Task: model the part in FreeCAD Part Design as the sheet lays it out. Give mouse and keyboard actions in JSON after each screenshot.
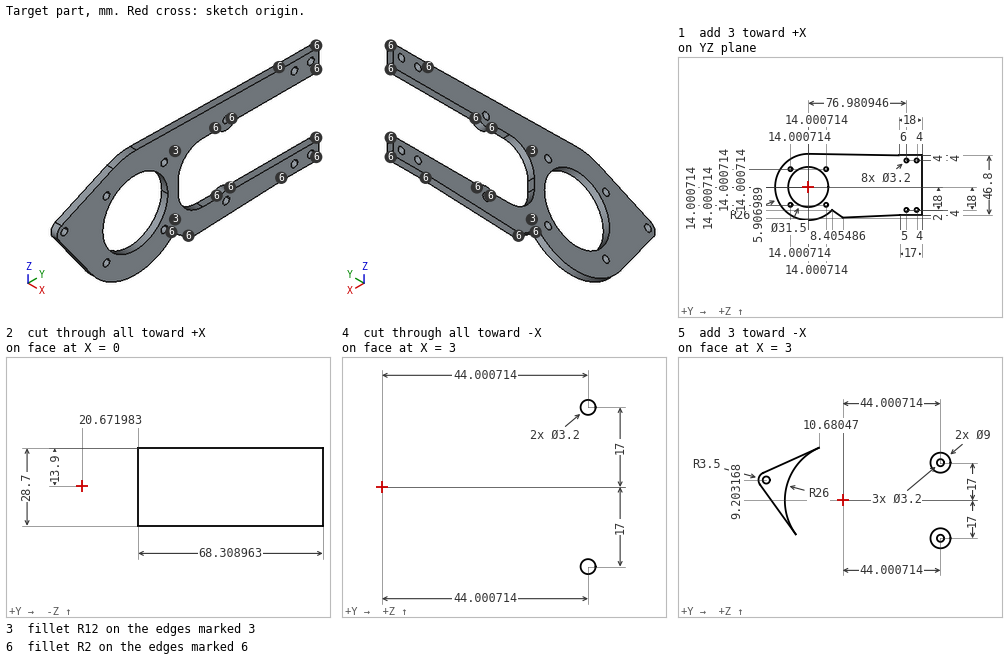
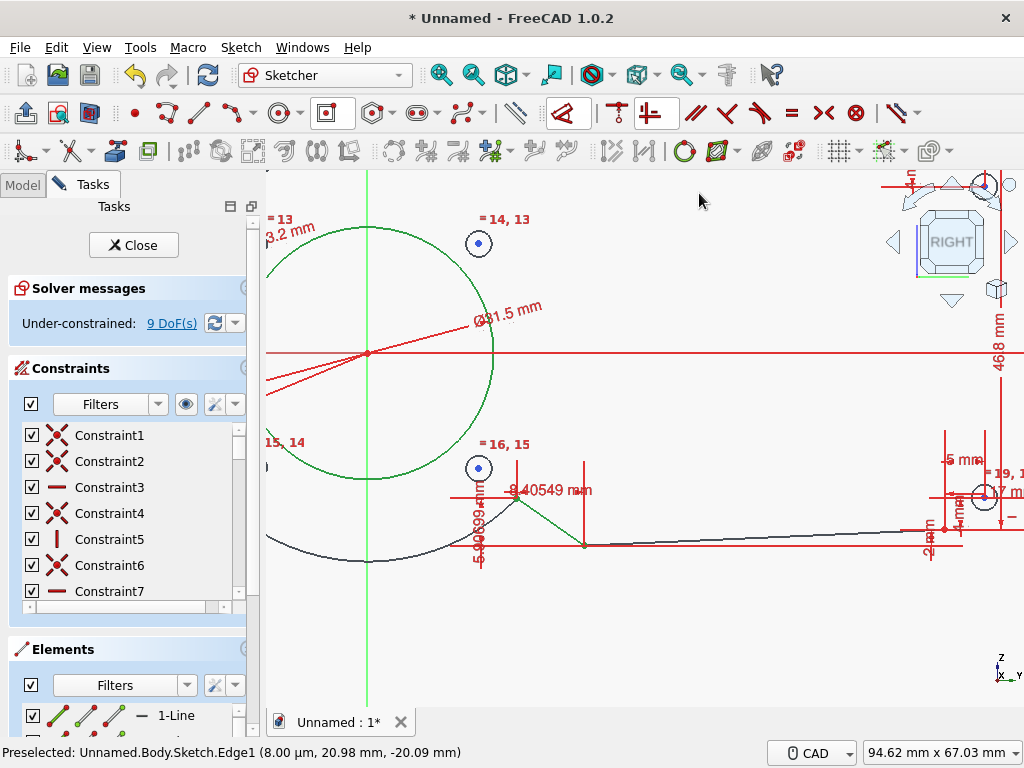
{"action": "scroll", "coordinate": [535, 514], "scroll_direction": "down", "scroll_amount": 4}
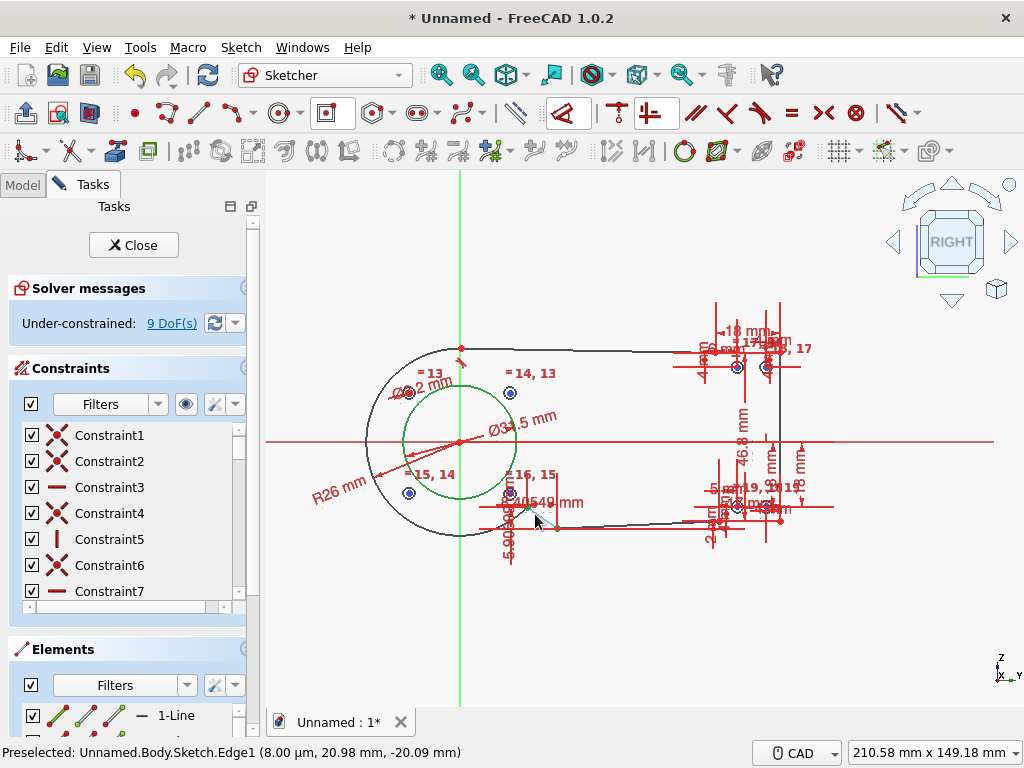
{"action": "left_click", "coordinate": [409, 393]}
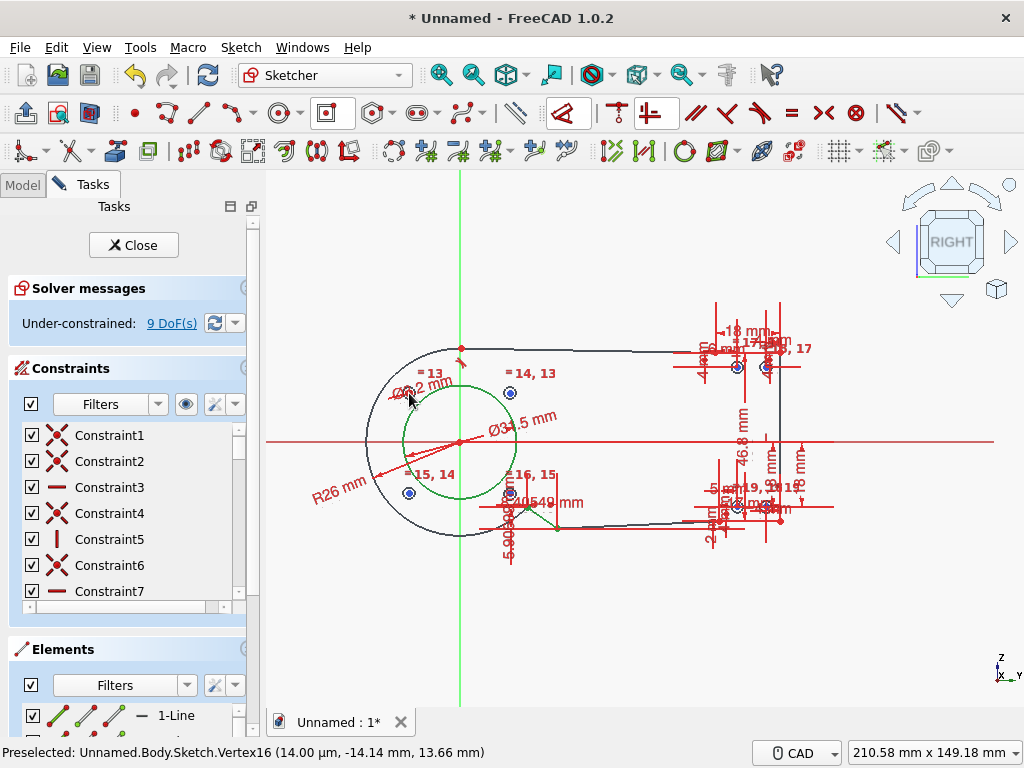
{"action": "left_click", "coordinate": [586, 114]}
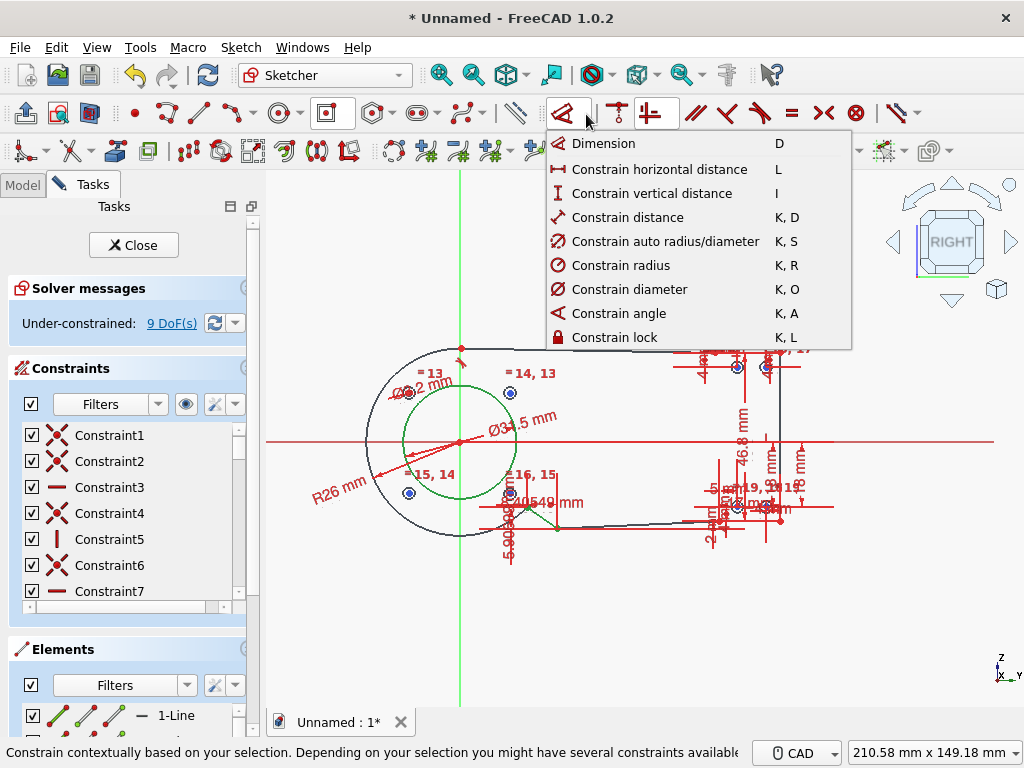
{"action": "left_click", "coordinate": [699, 169]}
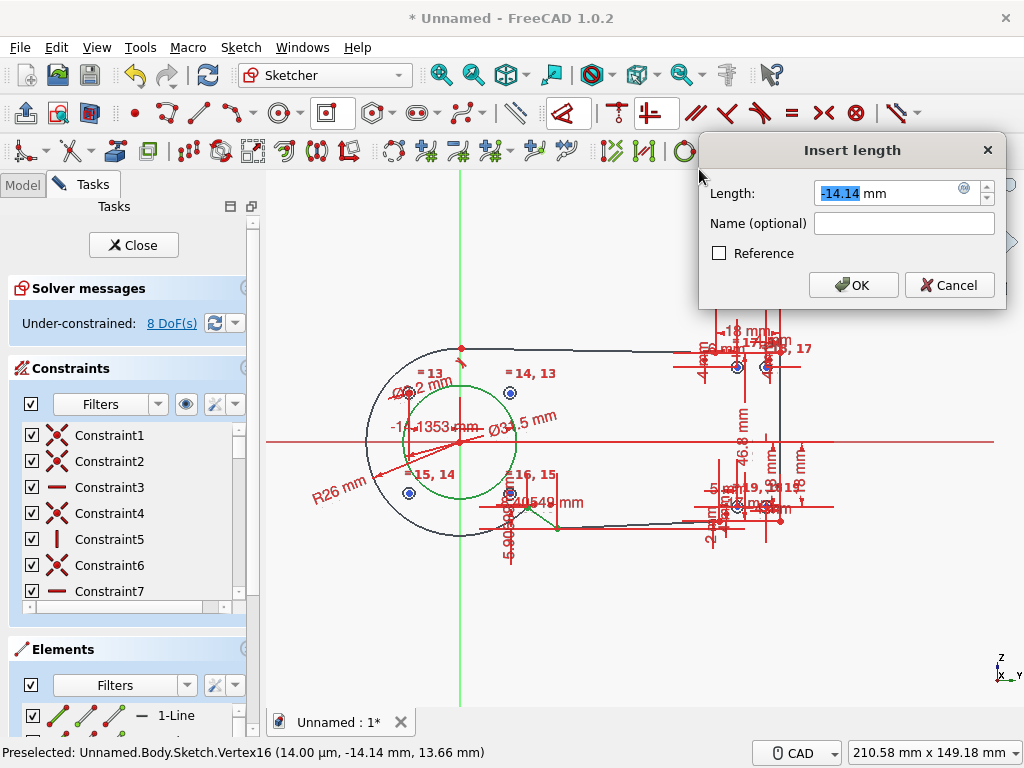
{"action": "type", "text": "-14.000714"}
{"action": "key", "text": "Return"}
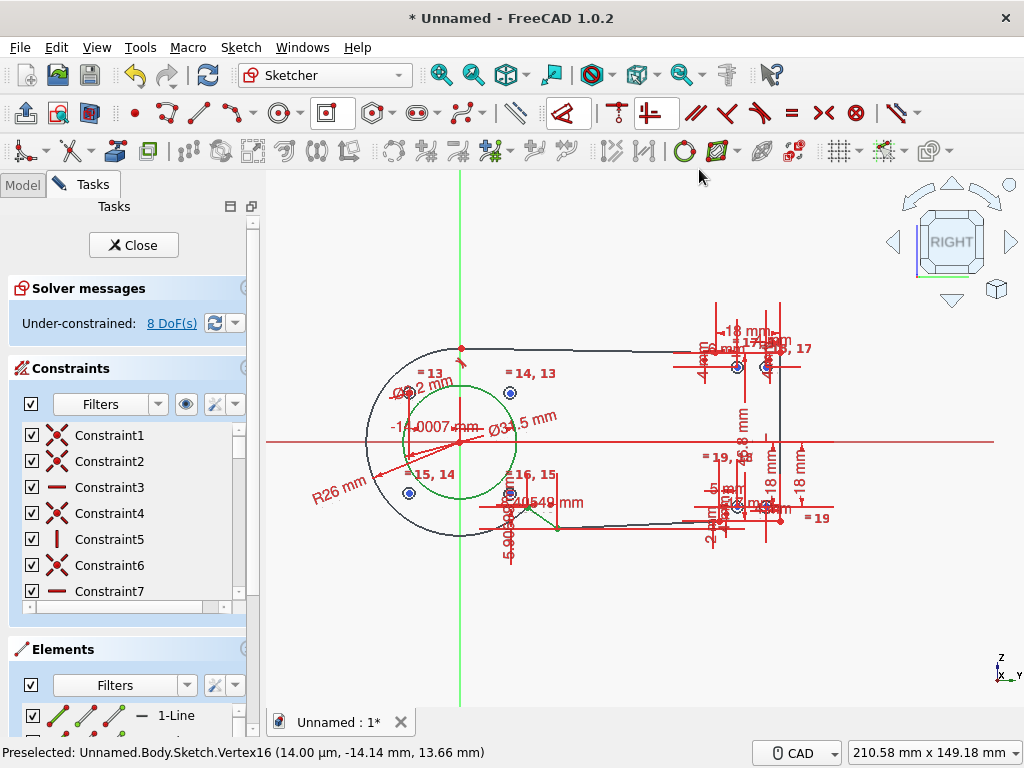
{"action": "left_click", "coordinate": [409, 393]}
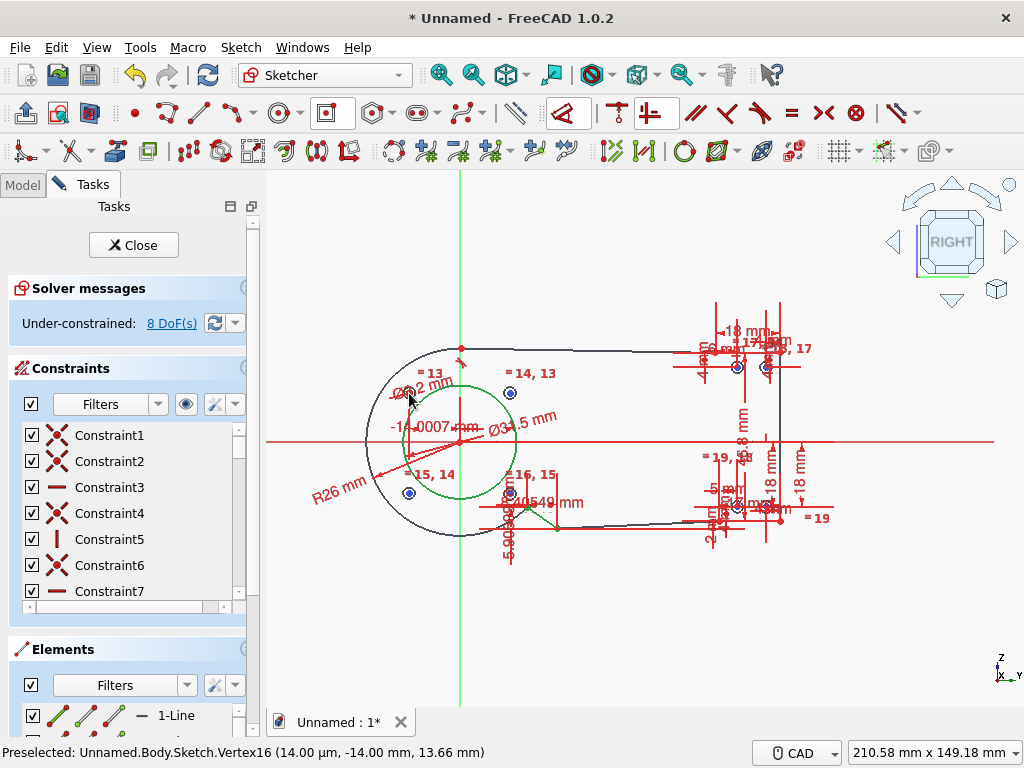
{"action": "key", "text": "i"}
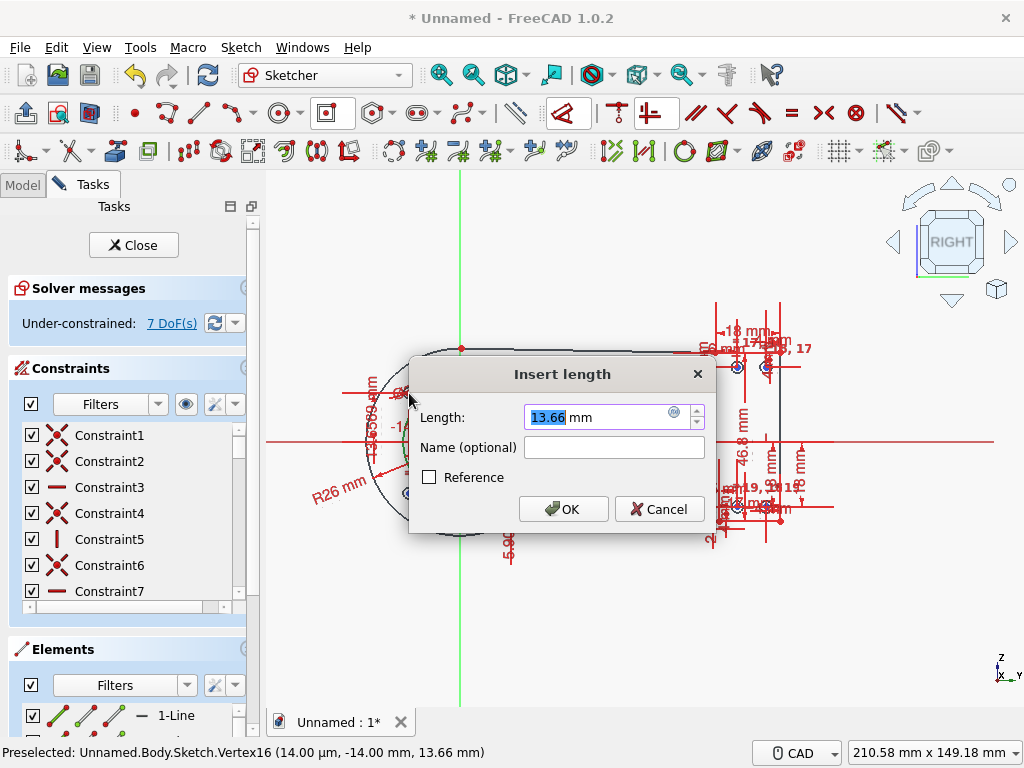
{"action": "type", "text": "14.000714"}
{"action": "key", "text": "Return"}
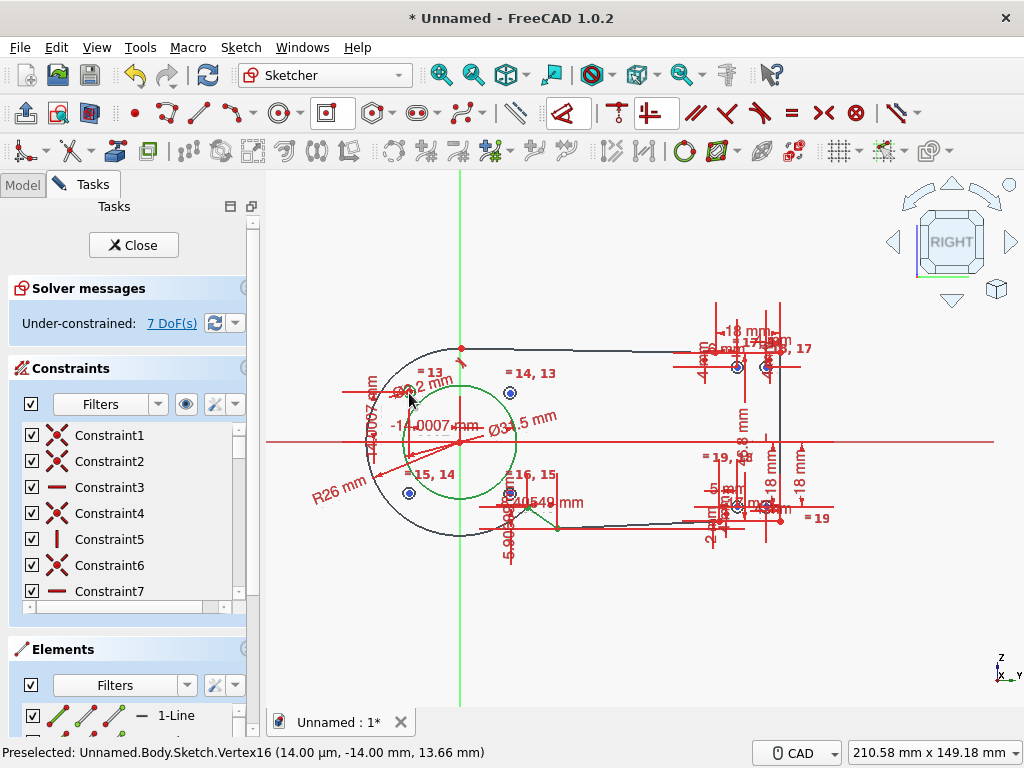
{"action": "left_click", "coordinate": [510, 393]}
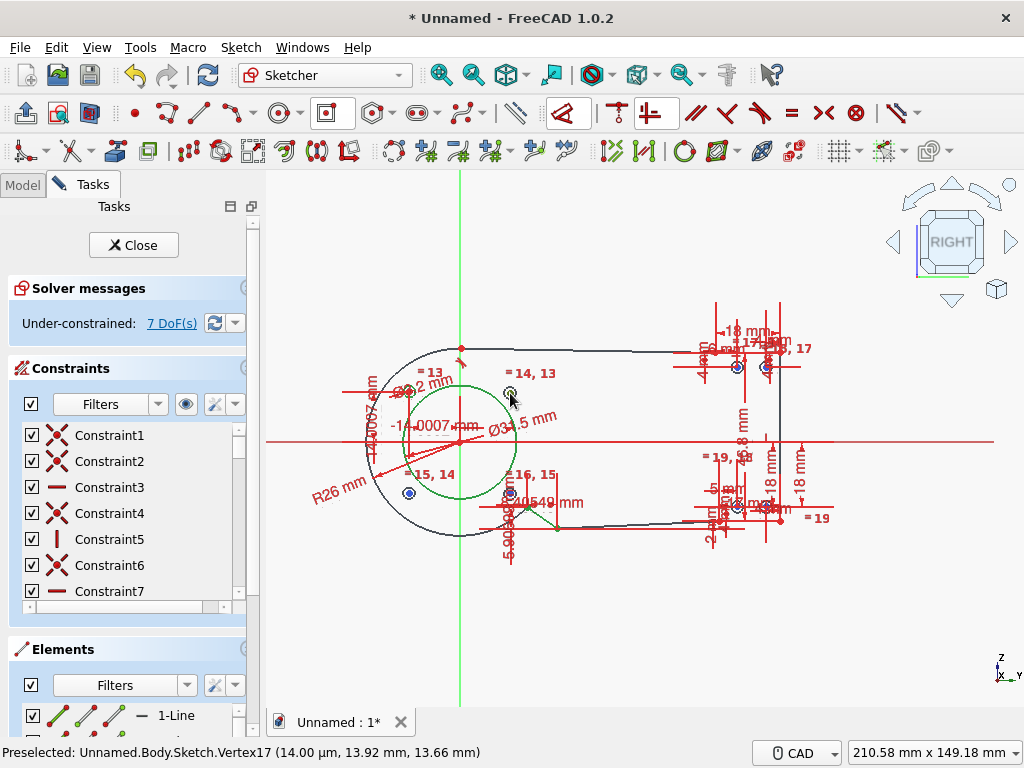
{"action": "left_click", "coordinate": [586, 114]}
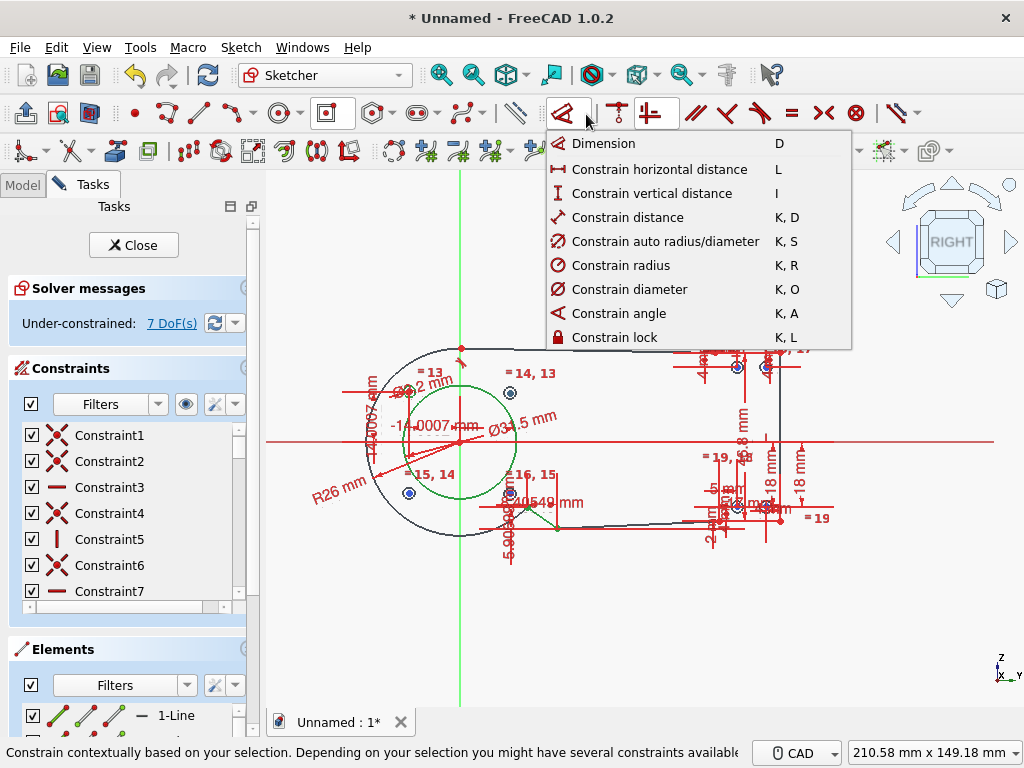
{"action": "left_click", "coordinate": [699, 169]}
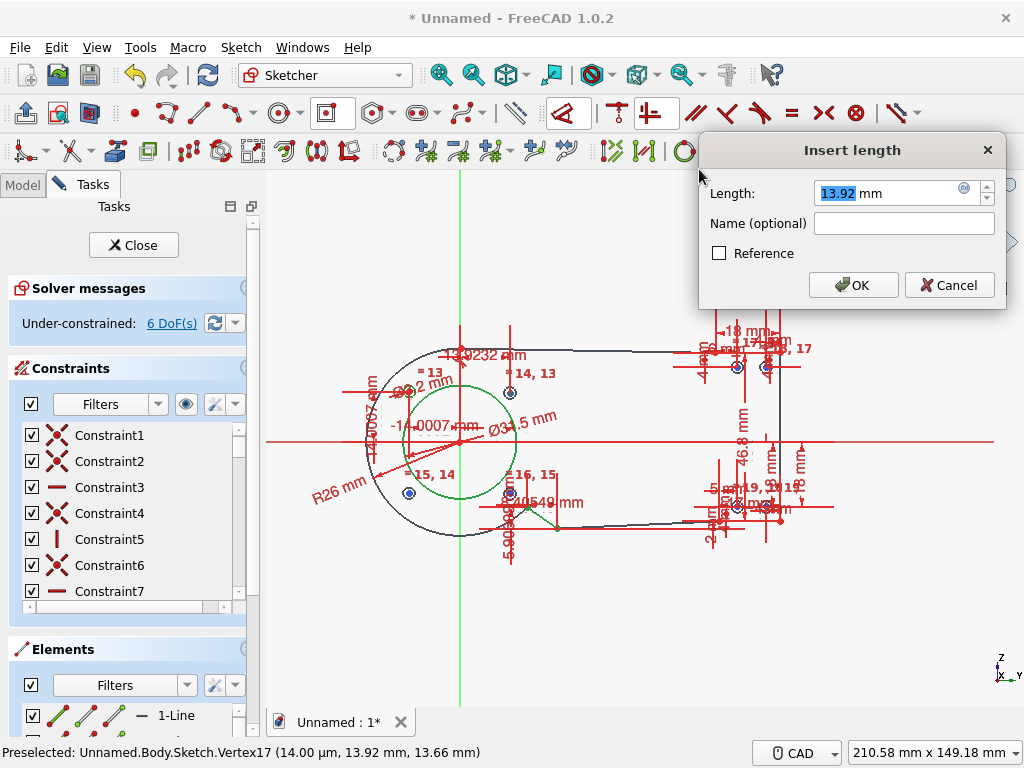
{"action": "type", "text": "14.000714"}
{"action": "key", "text": "Return"}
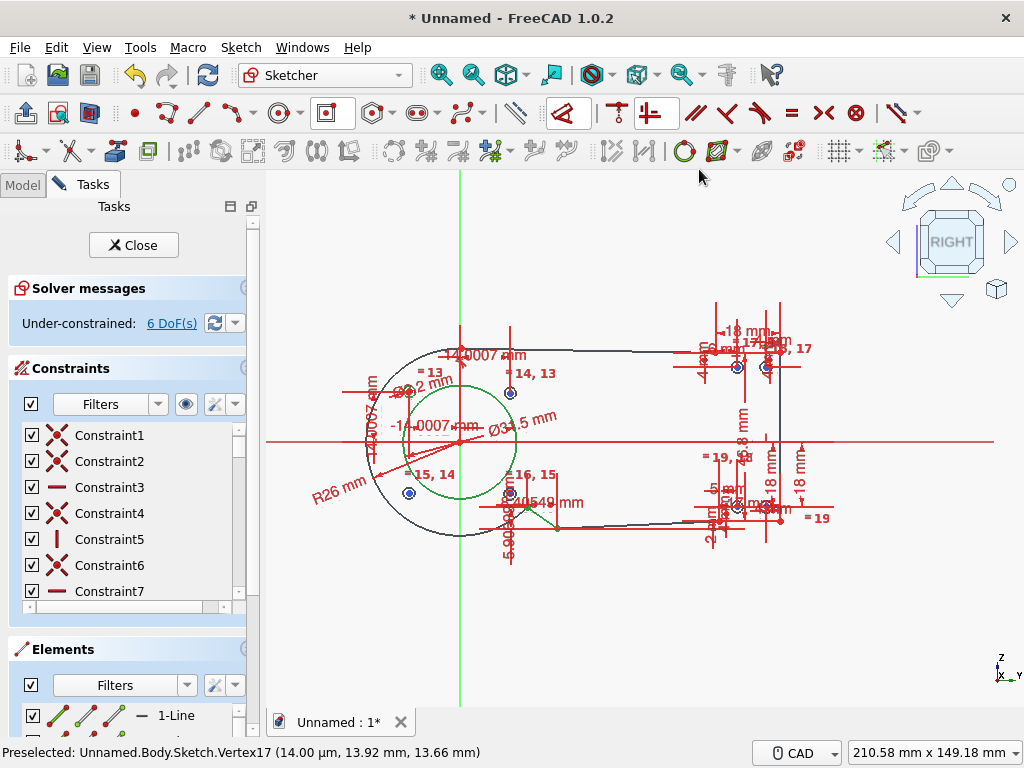
{"action": "left_click", "coordinate": [510, 393]}